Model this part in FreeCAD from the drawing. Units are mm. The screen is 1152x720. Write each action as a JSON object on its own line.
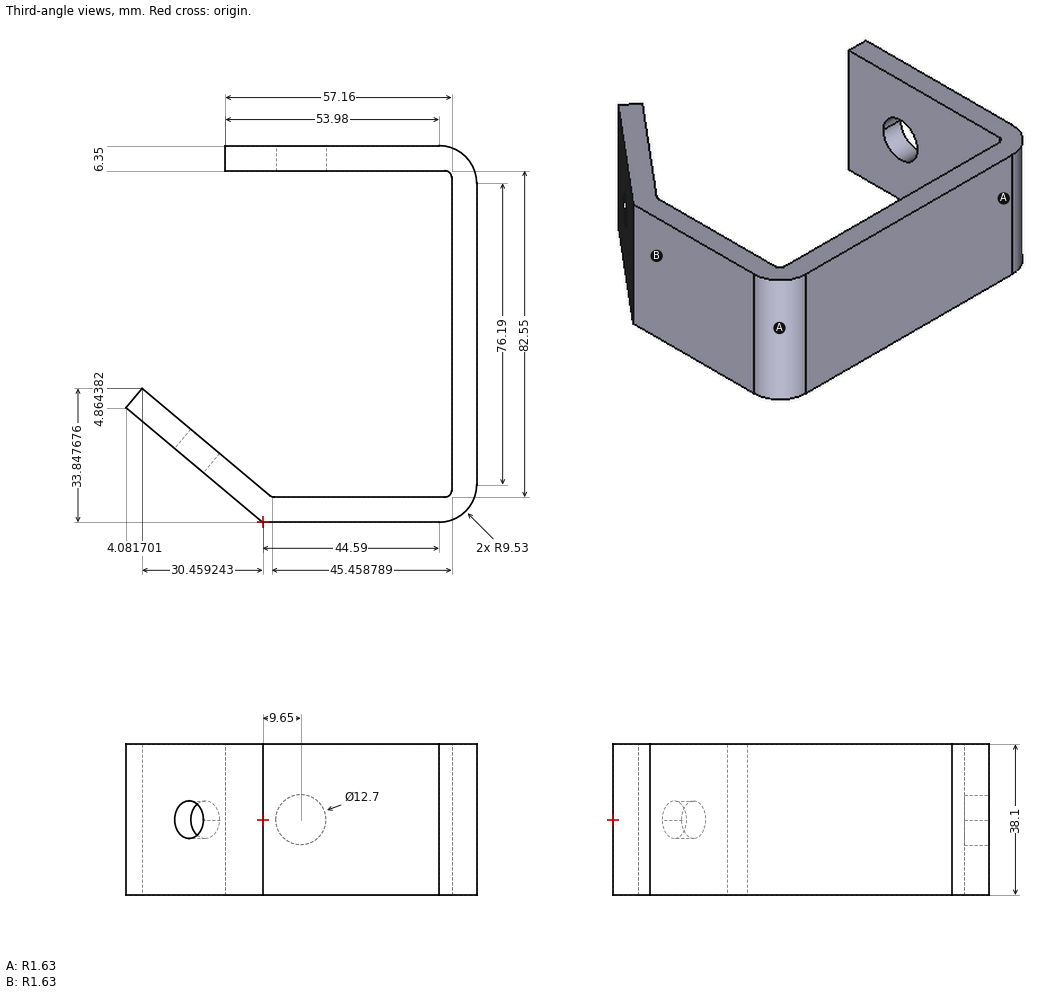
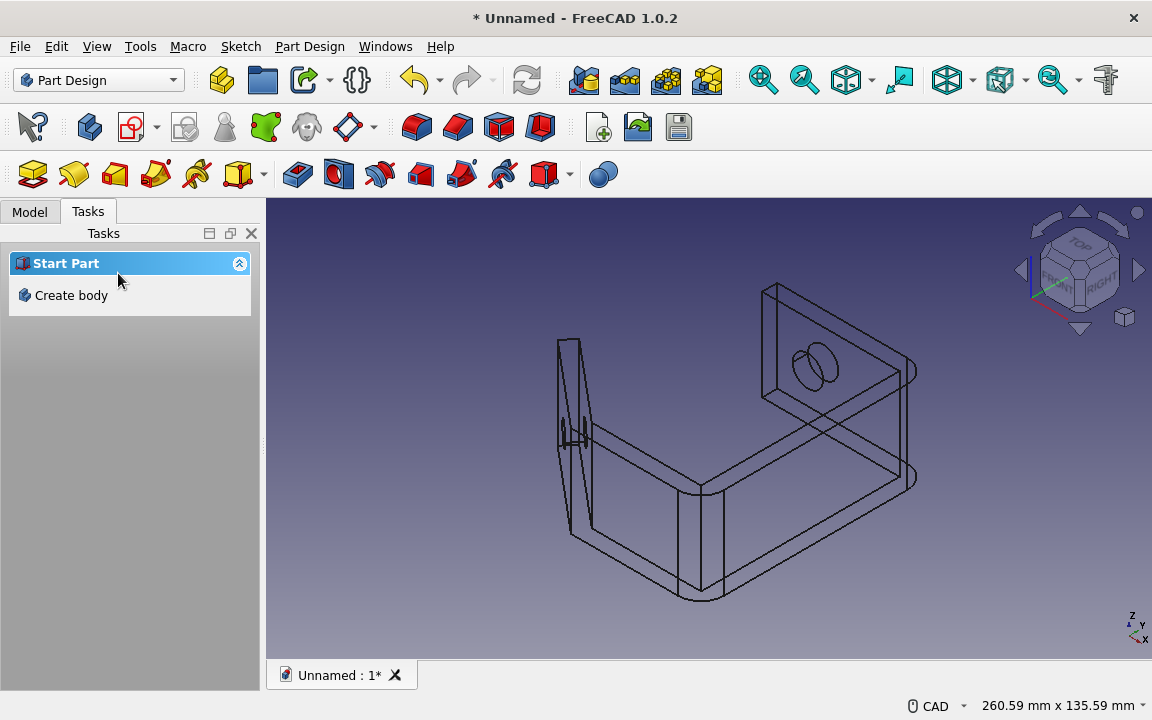
{"action": "left_click", "coordinate": [701, 538]}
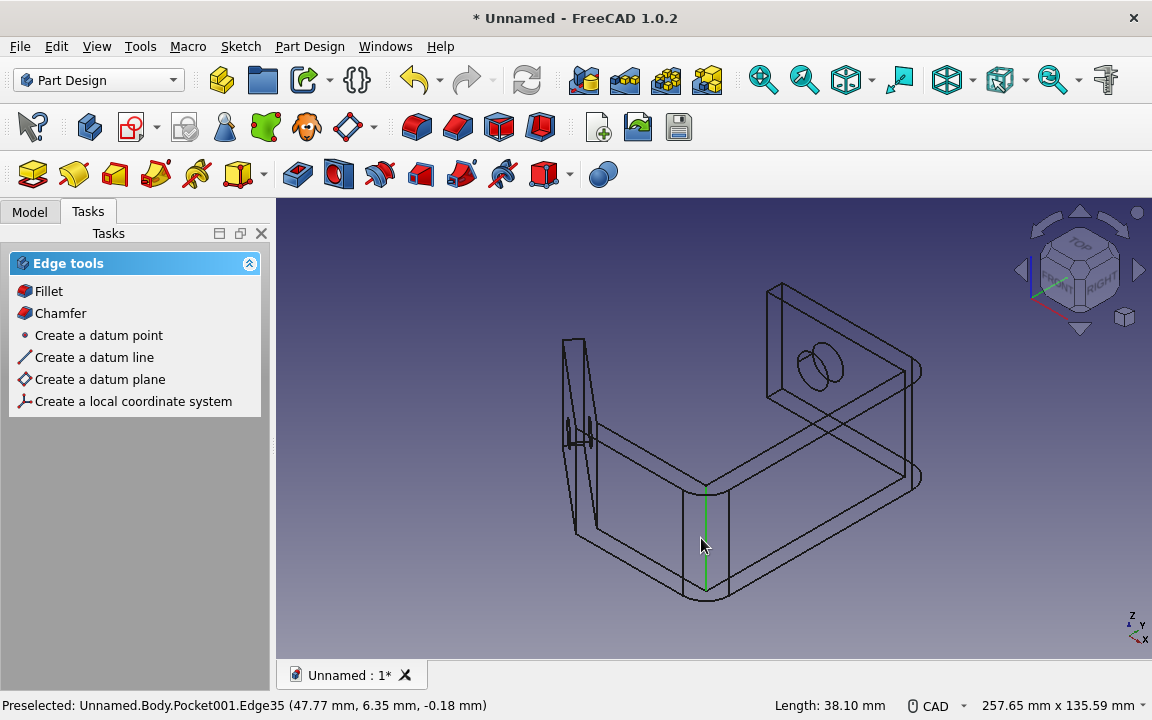
{"action": "left_click", "coordinate": [905, 423], "text": "ctrl"}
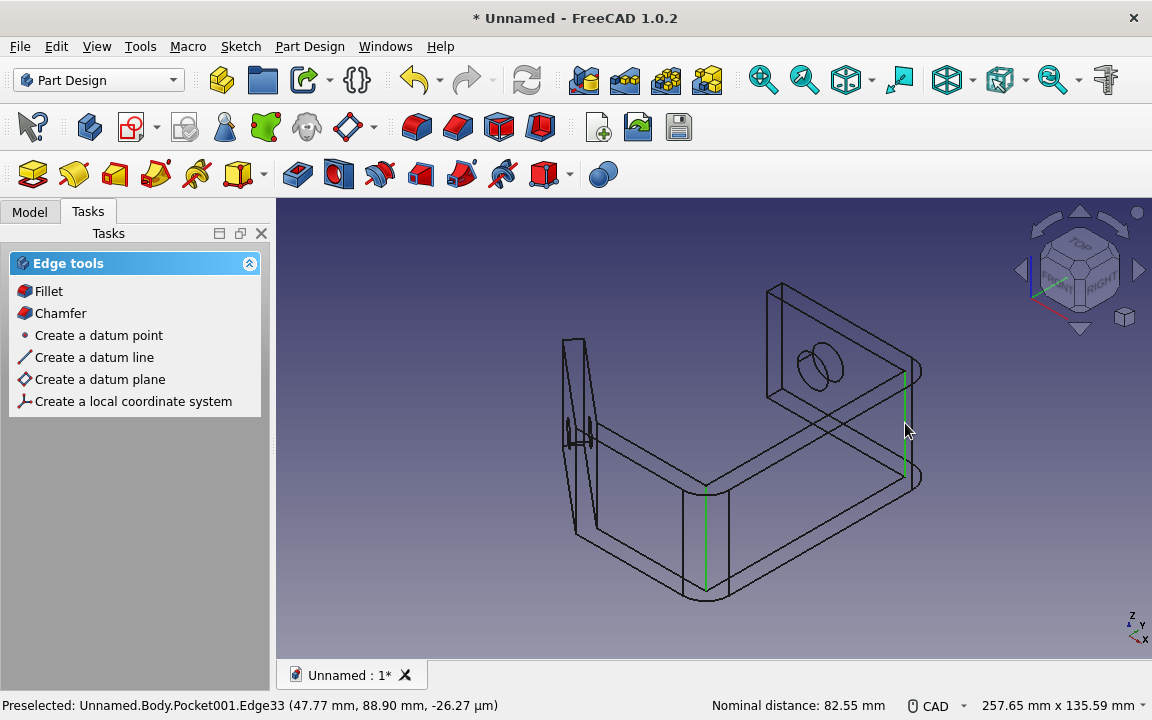
{"action": "key", "text": "v 1"}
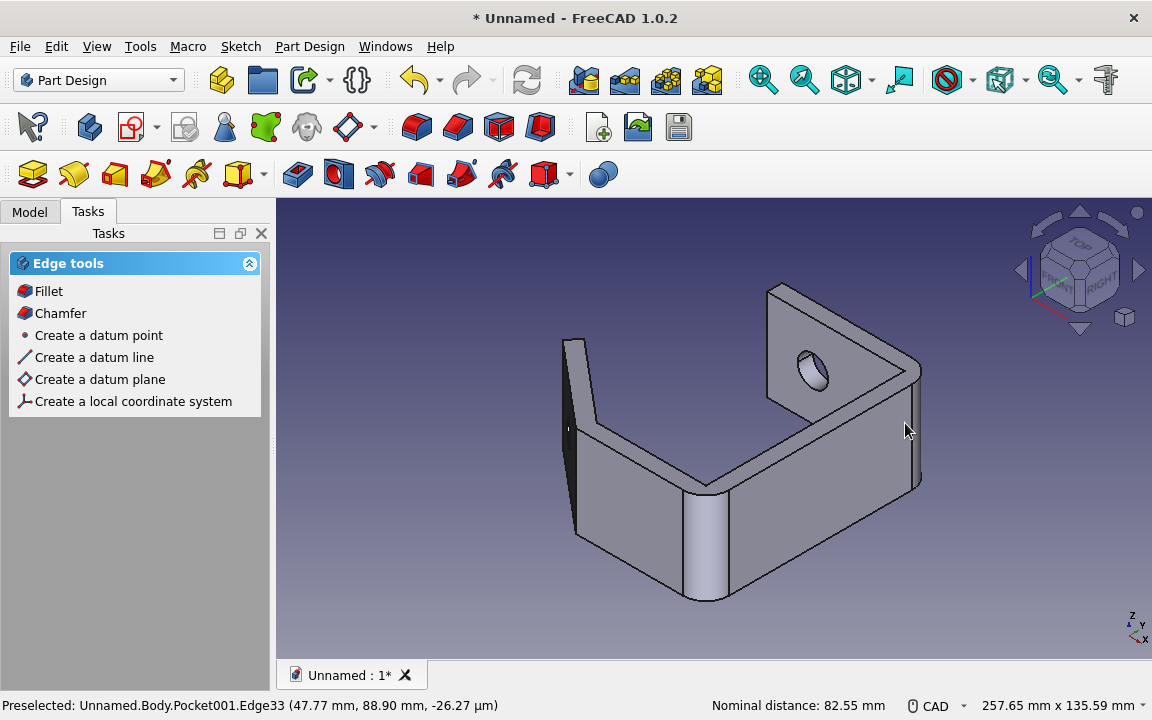
{"action": "left_click", "coordinate": [417, 128]}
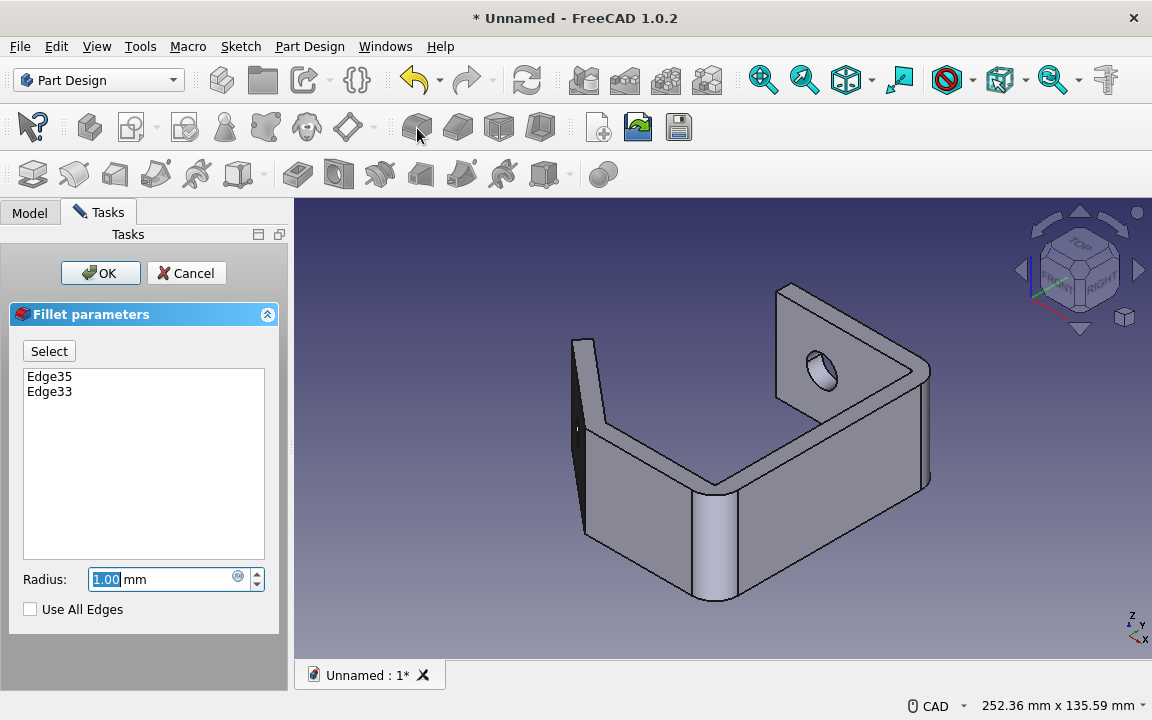
{"action": "type", "text": "1.63"}
{"action": "key", "text": "Tab"}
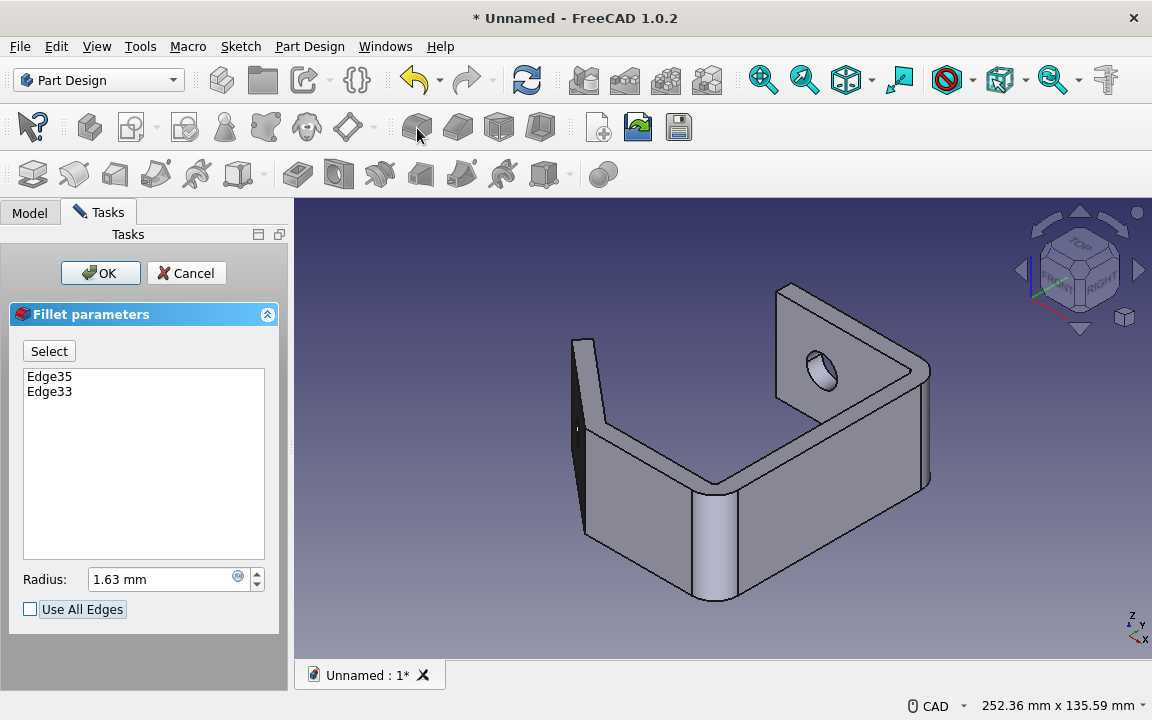
{"action": "left_click", "coordinate": [101, 273]}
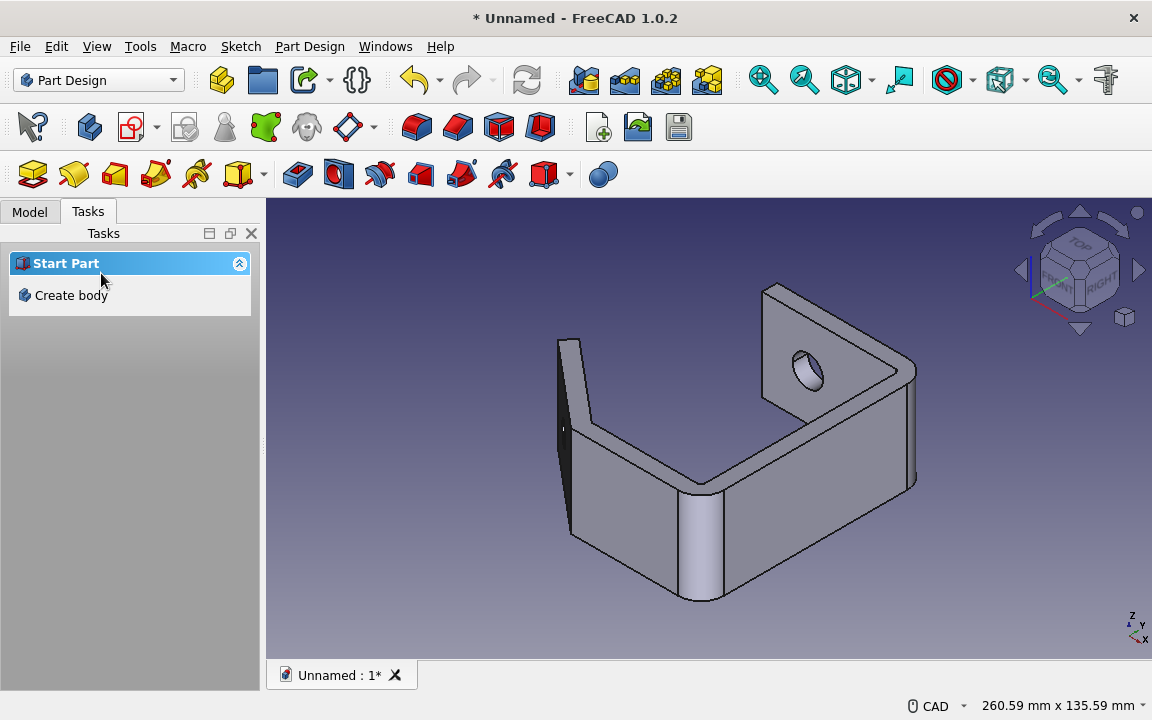
{"action": "key", "text": "2"}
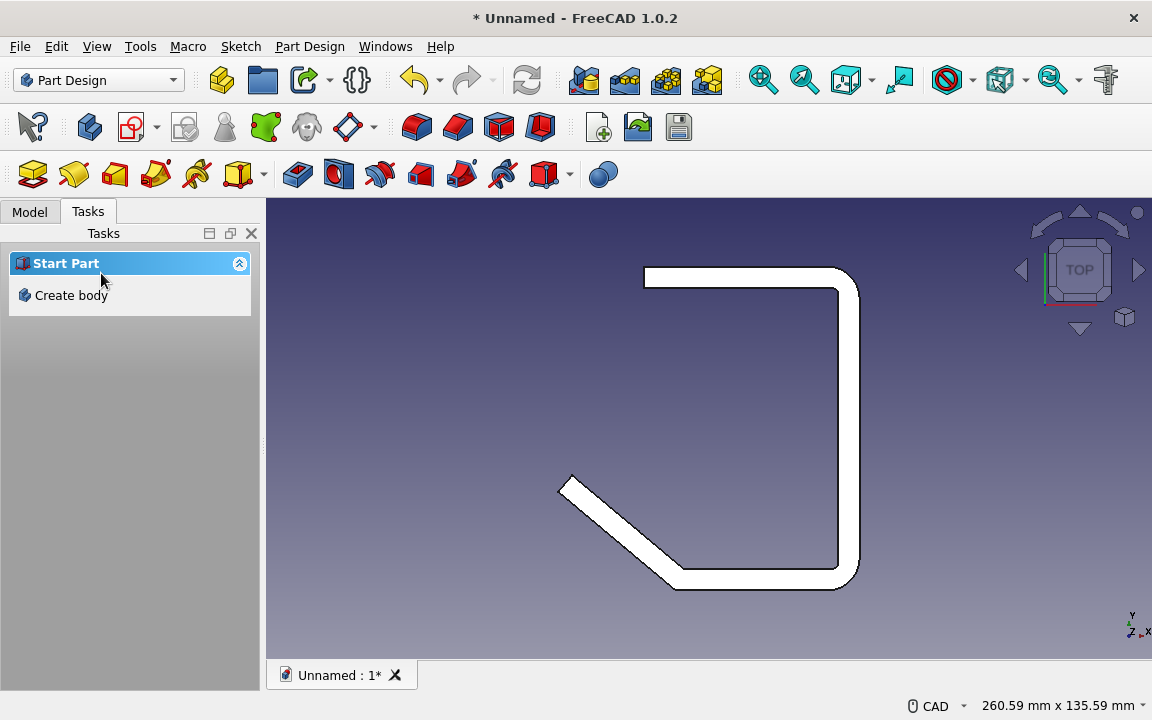
{"action": "key", "text": "0"}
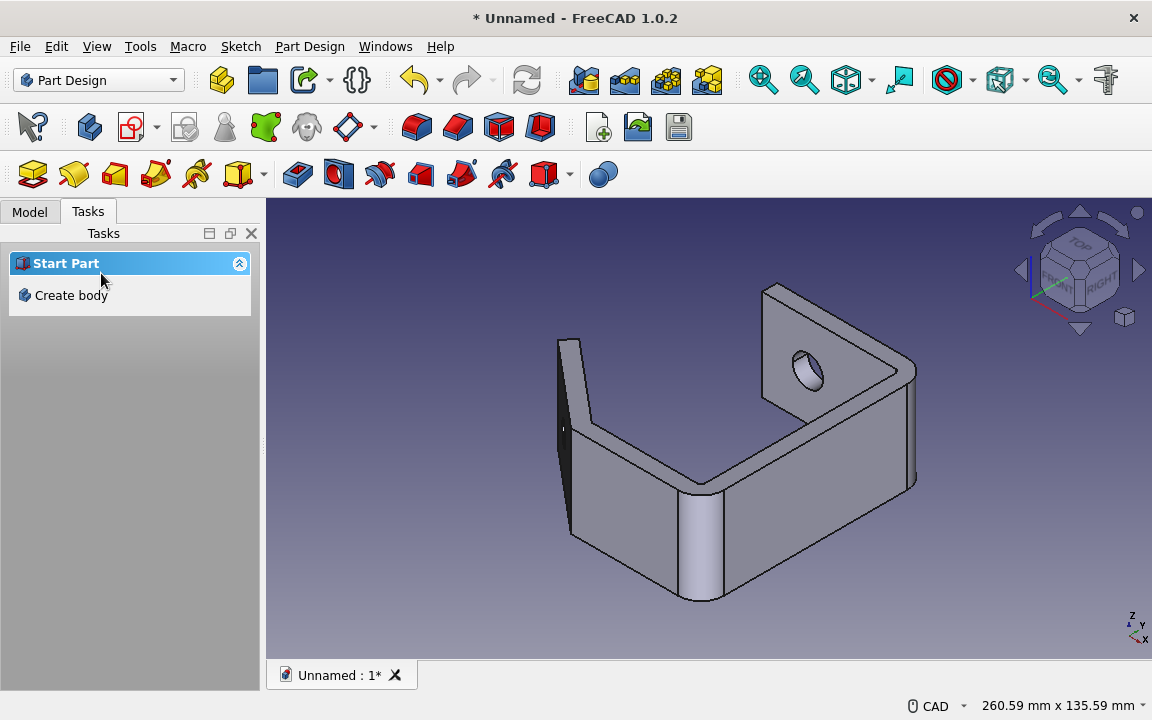
{"action": "key", "text": "1"}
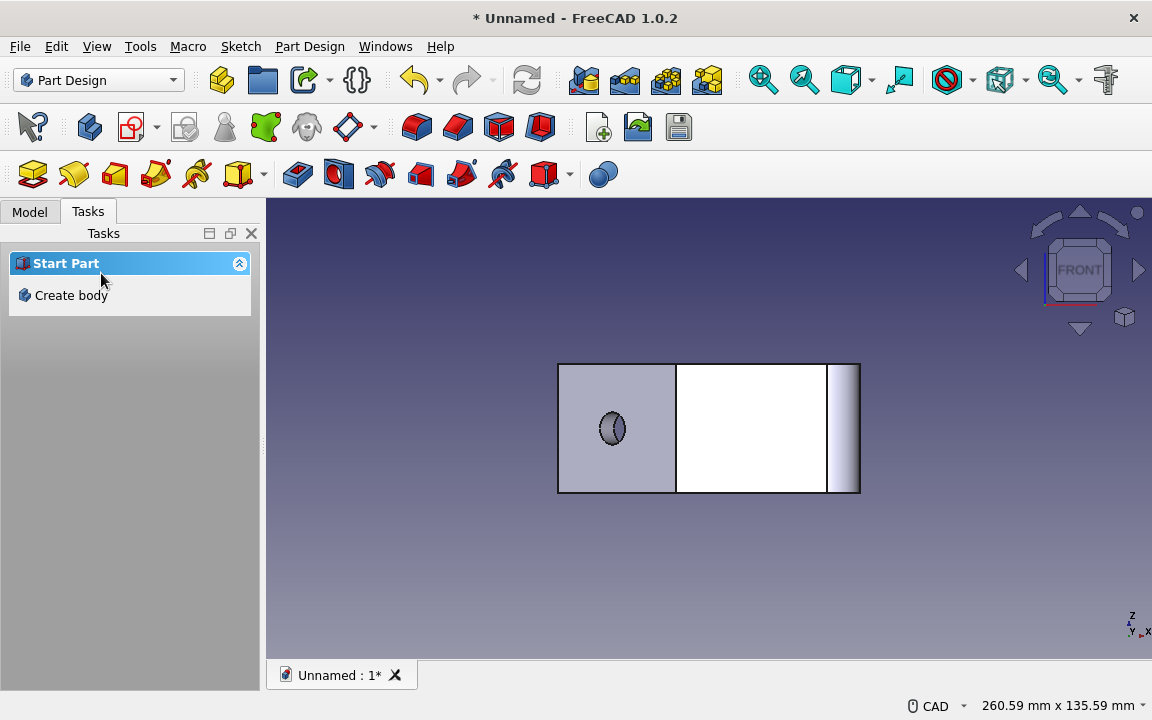
{"action": "left_click", "coordinate": [764, 80]}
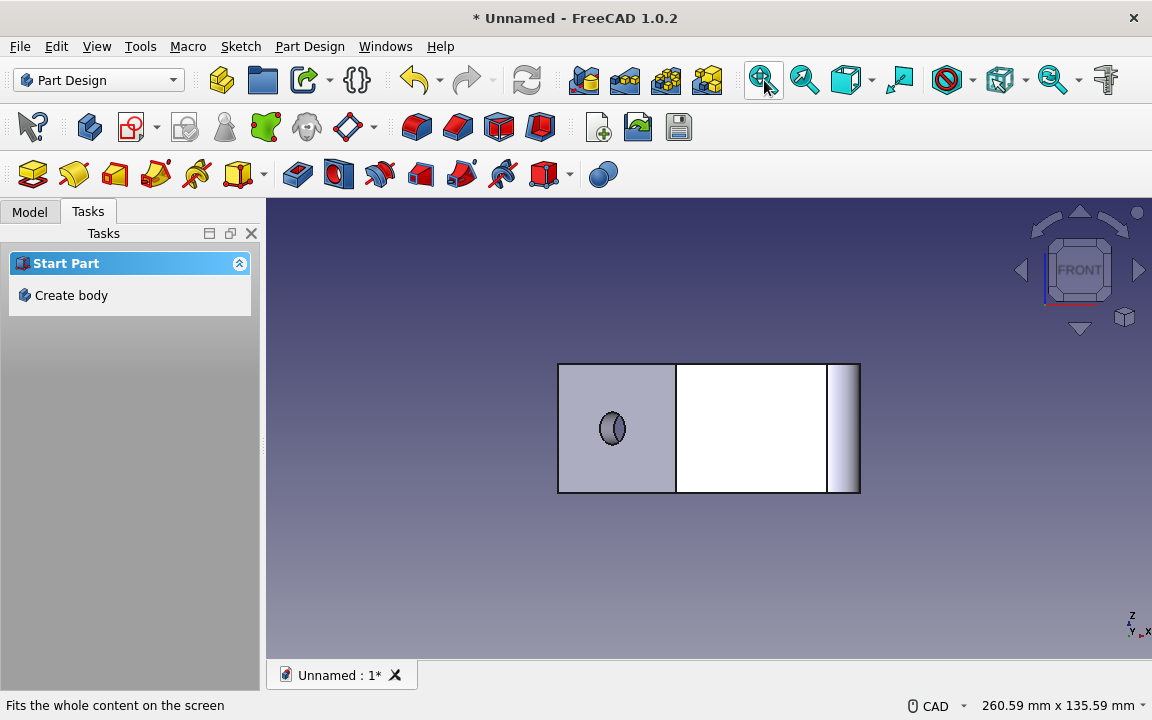
{"action": "key", "text": "3"}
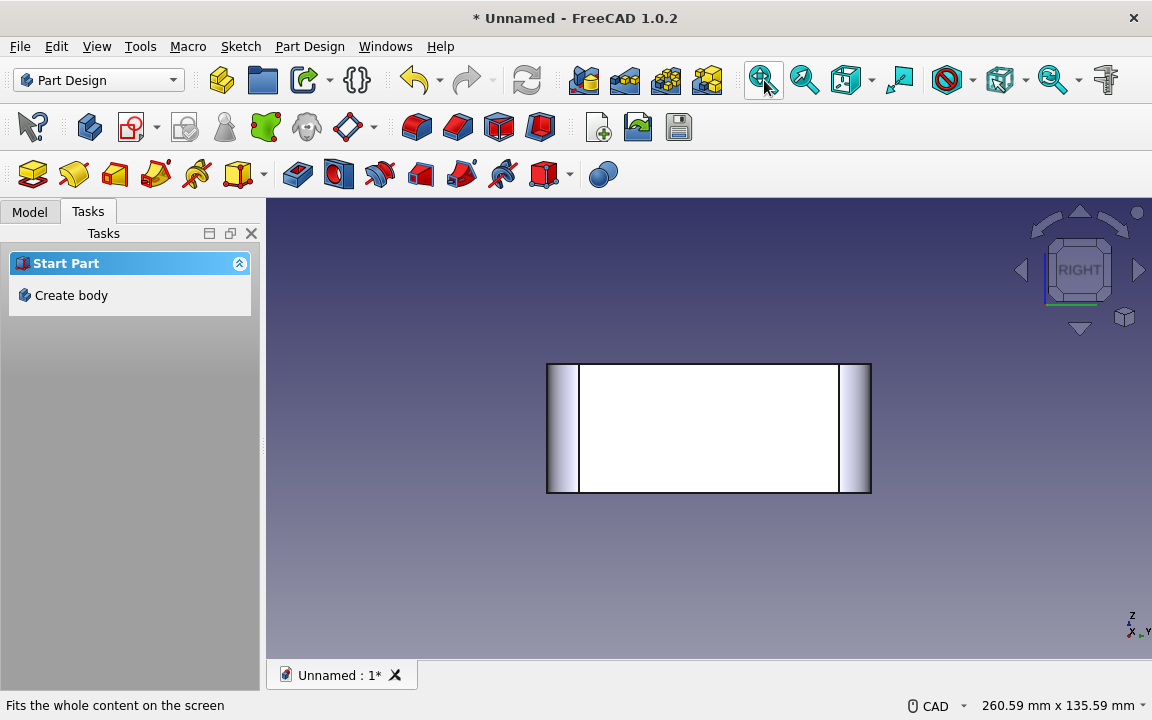
{"action": "left_click", "coordinate": [764, 80]}